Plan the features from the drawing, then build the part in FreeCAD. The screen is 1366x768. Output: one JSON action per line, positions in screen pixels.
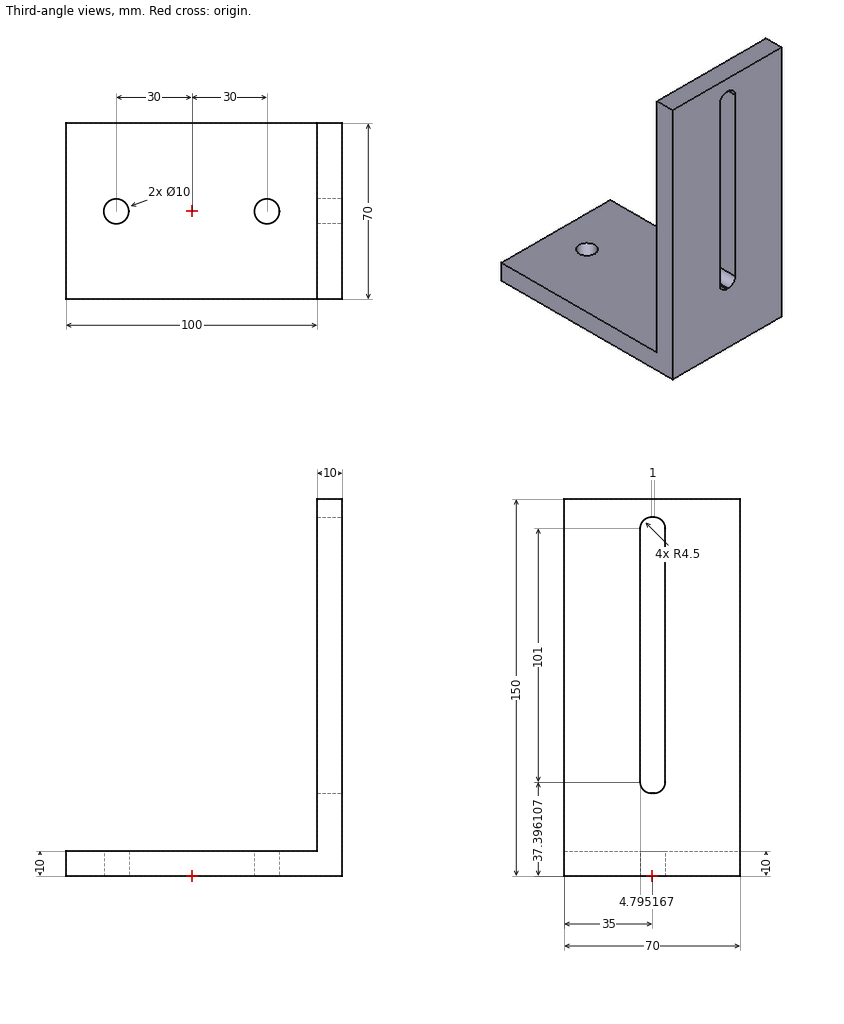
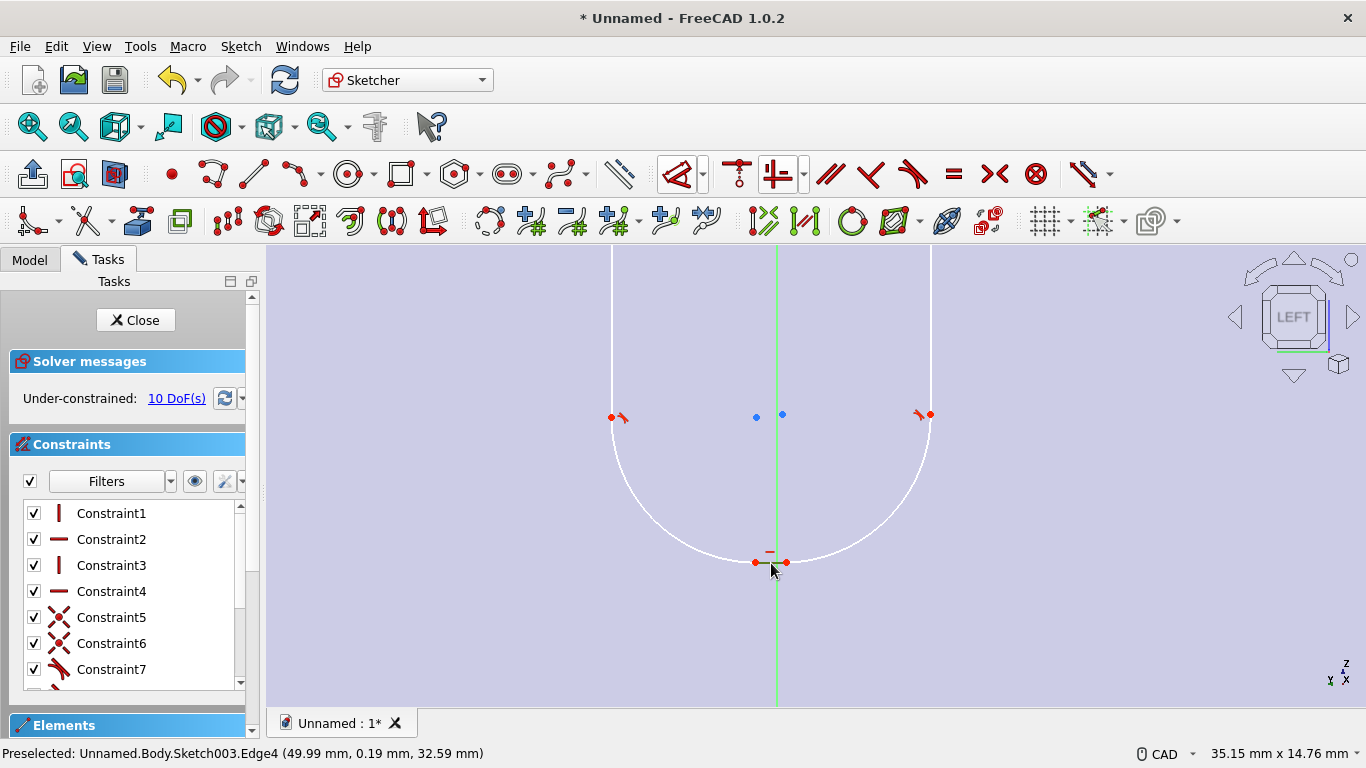
{"action": "scroll", "coordinate": [746, 549], "scroll_direction": "down", "scroll_amount": 14}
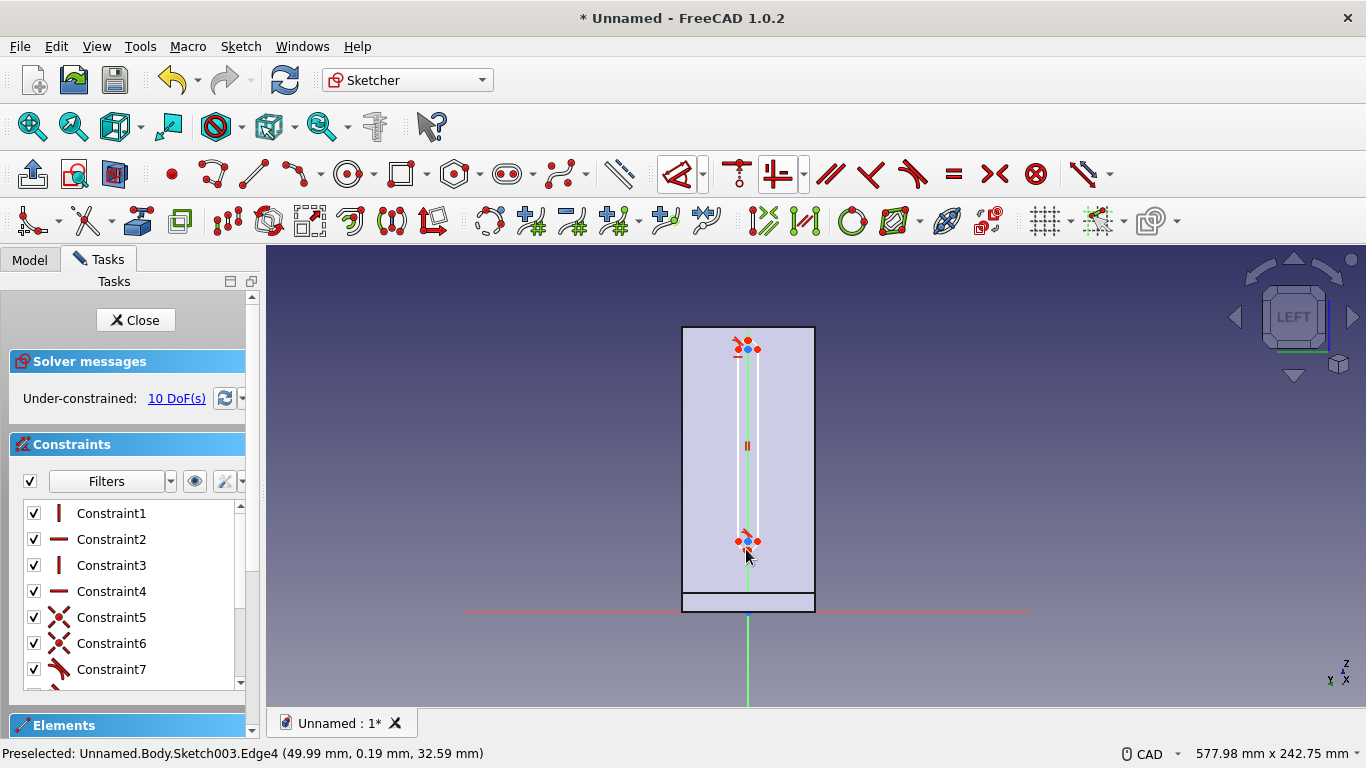
{"action": "scroll", "coordinate": [739, 546], "scroll_direction": "up", "scroll_amount": 7}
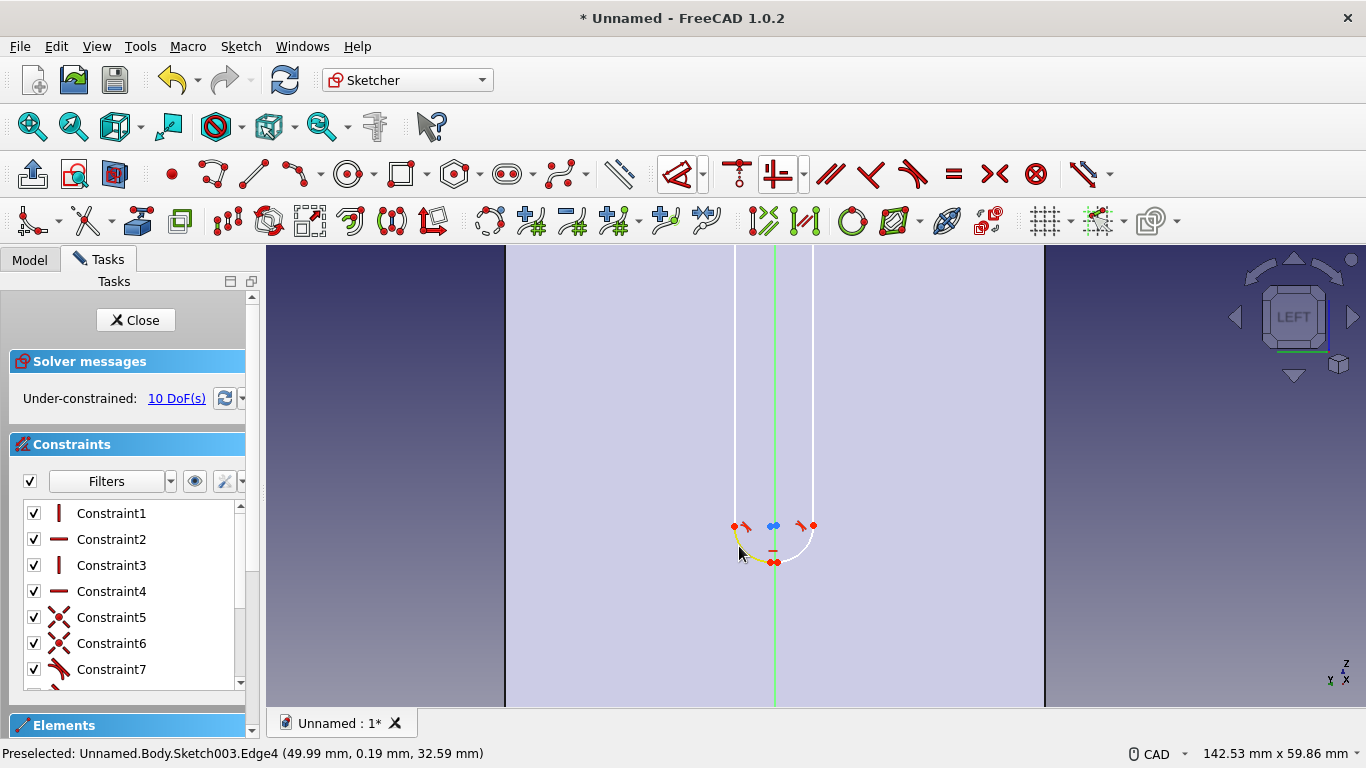
{"action": "left_click", "coordinate": [738, 542]}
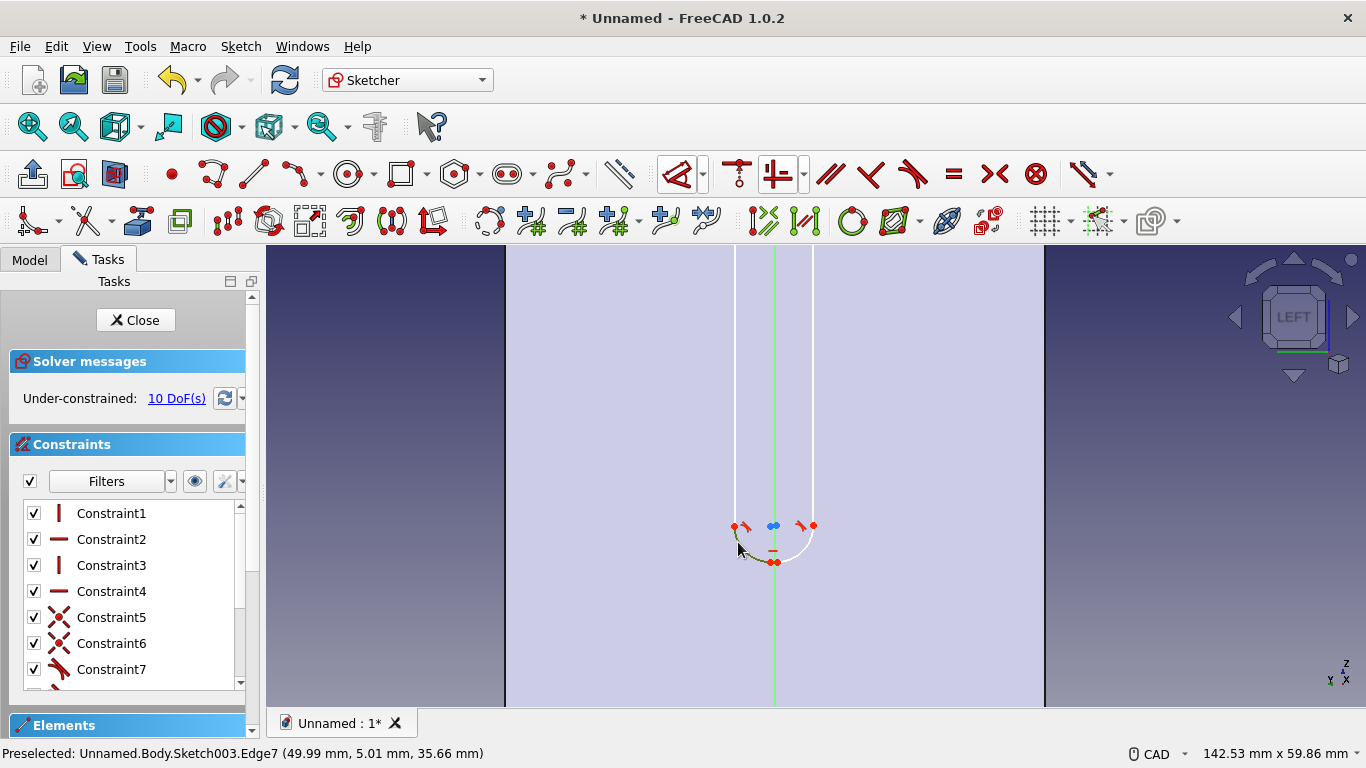
{"action": "left_click", "coordinate": [913, 174]}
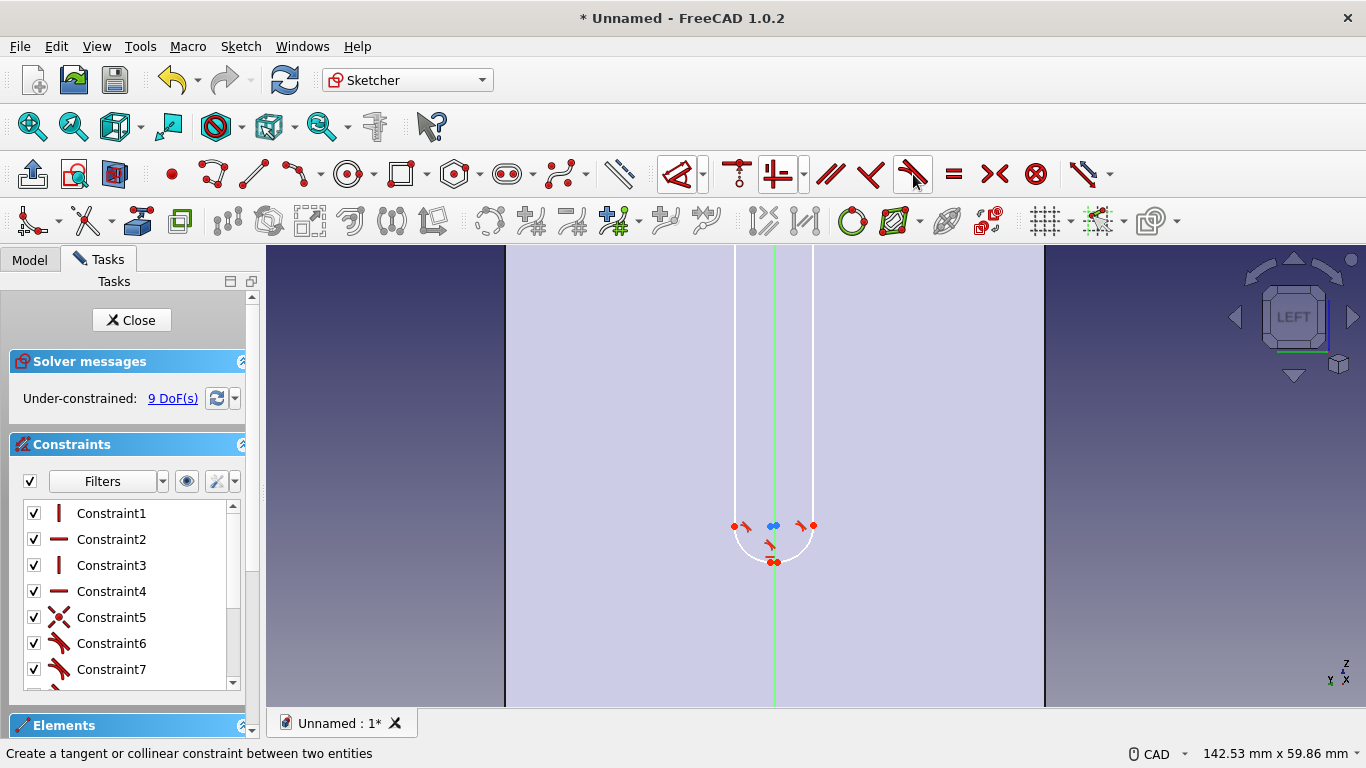
{"action": "scroll", "coordinate": [774, 562], "scroll_direction": "up", "scroll_amount": 7}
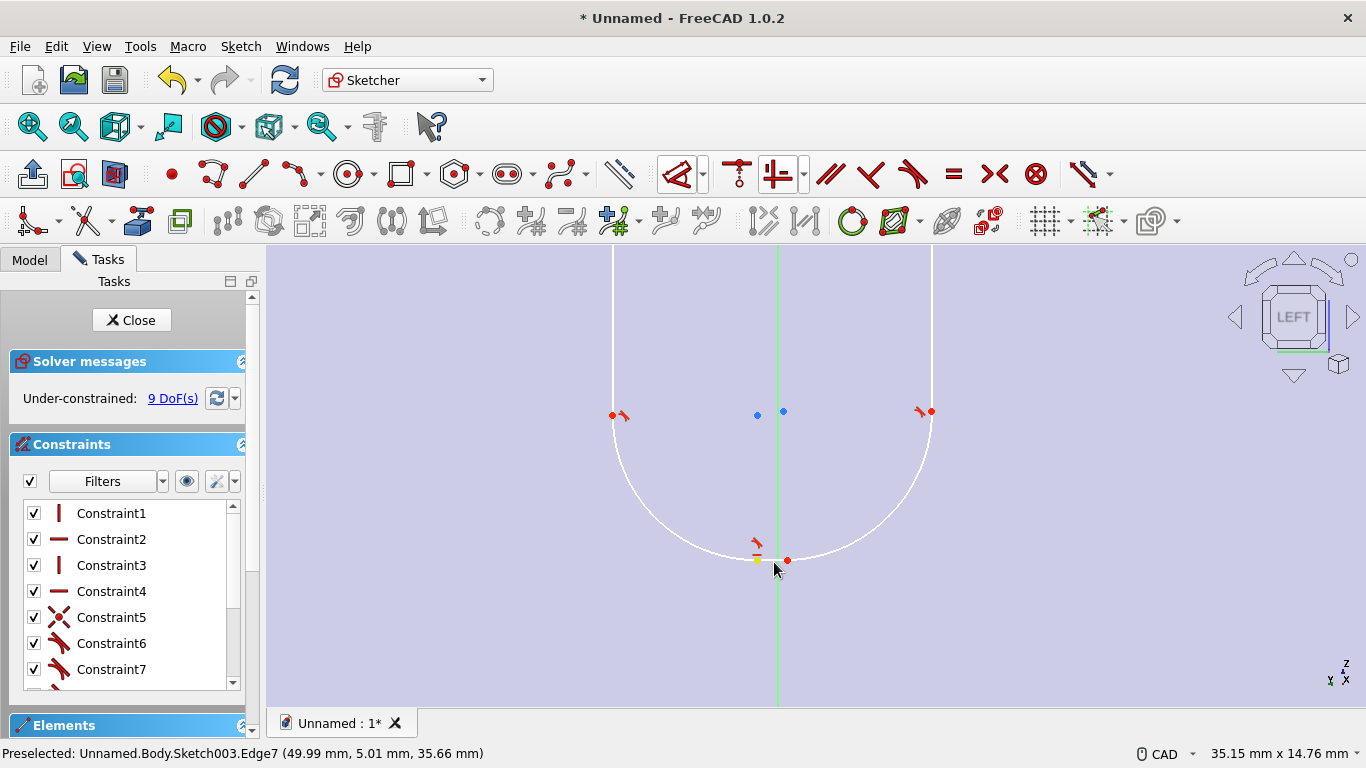
{"action": "left_click", "coordinate": [773, 560]}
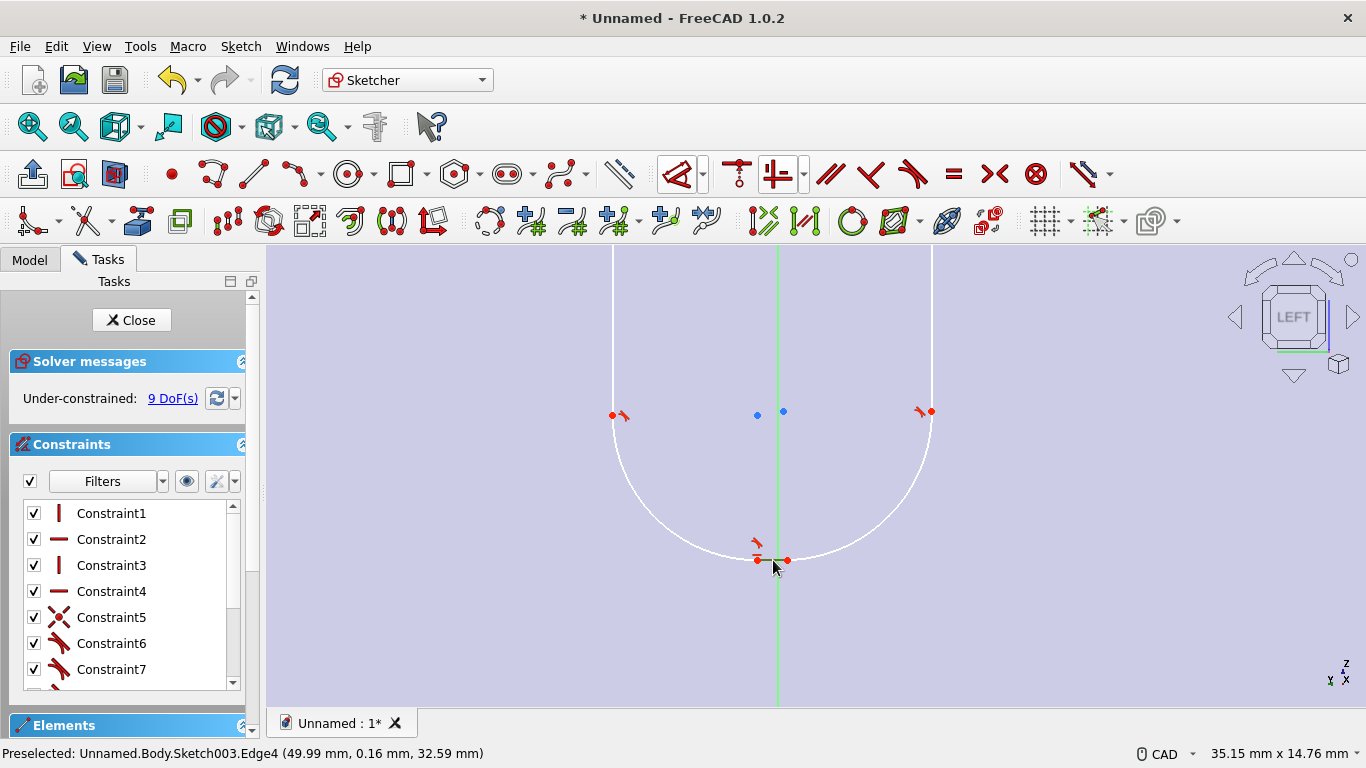
{"action": "scroll", "coordinate": [746, 549], "scroll_direction": "down", "scroll_amount": 14}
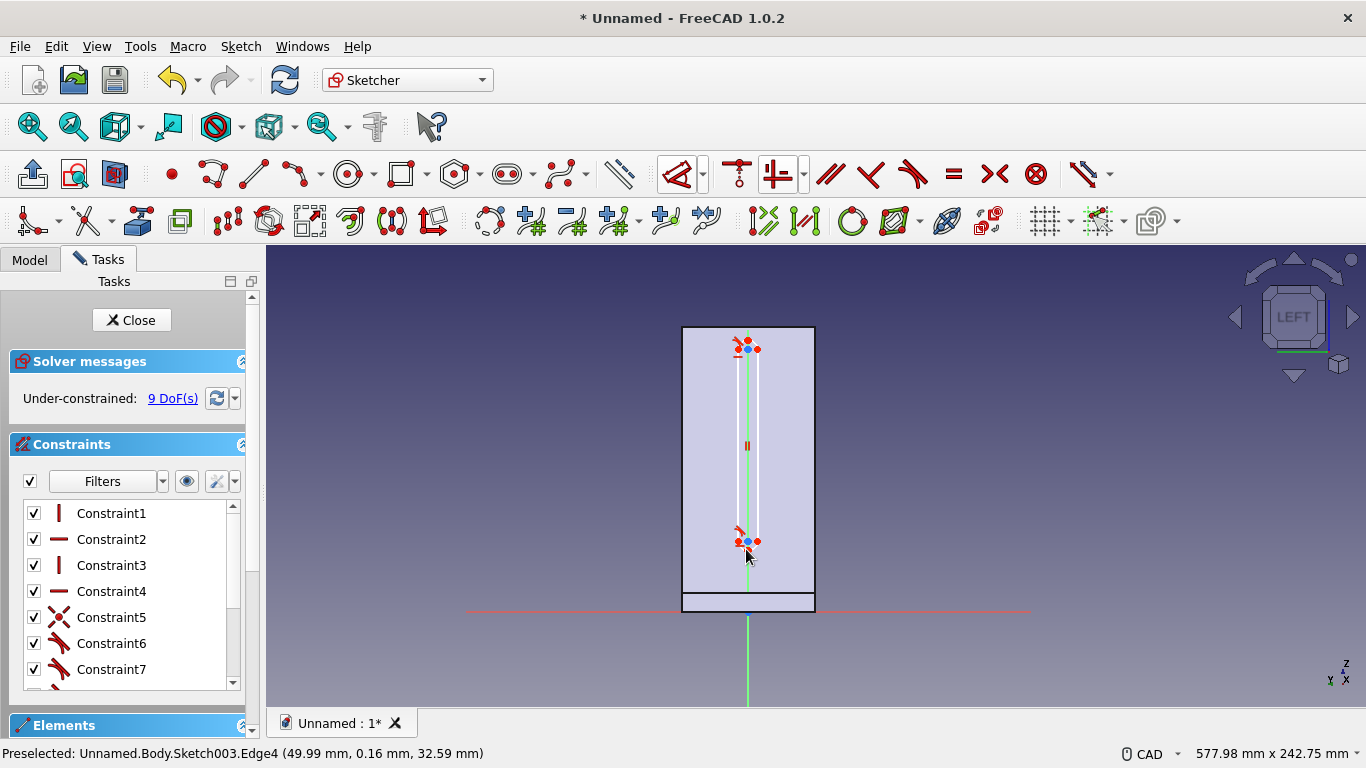
{"action": "scroll", "coordinate": [753, 549], "scroll_direction": "up", "scroll_amount": 7}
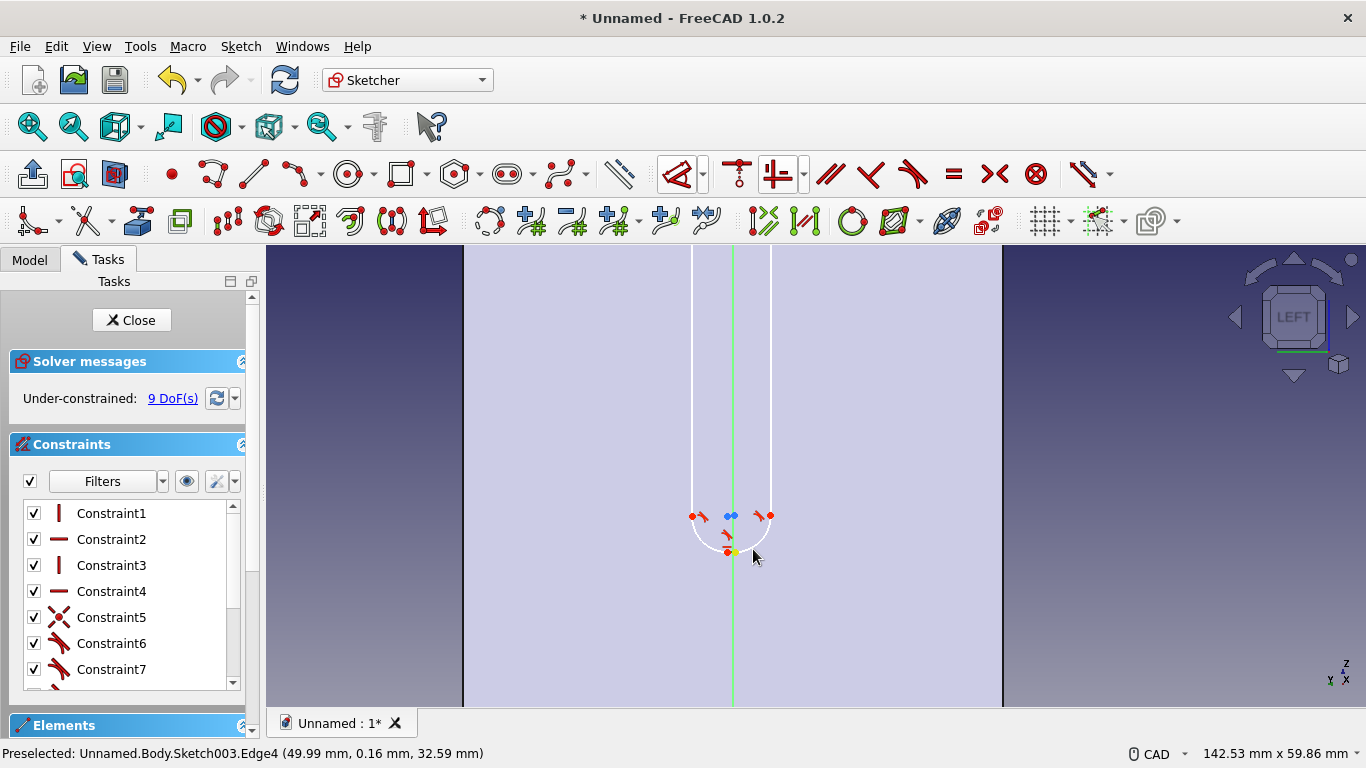
{"action": "left_click", "coordinate": [751, 548]}